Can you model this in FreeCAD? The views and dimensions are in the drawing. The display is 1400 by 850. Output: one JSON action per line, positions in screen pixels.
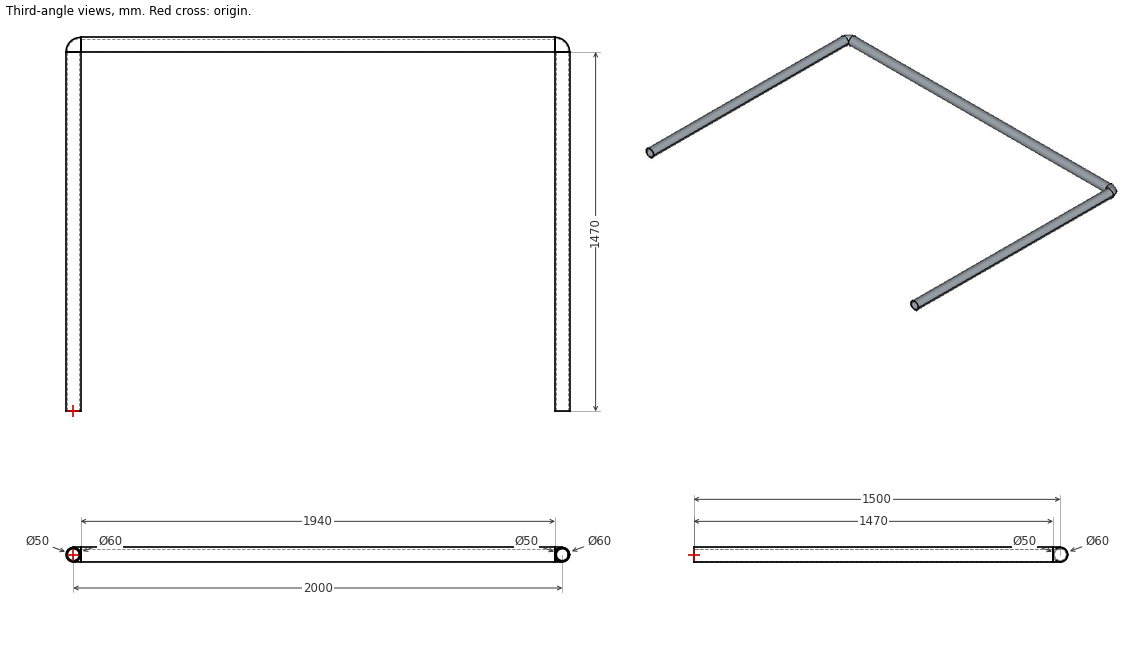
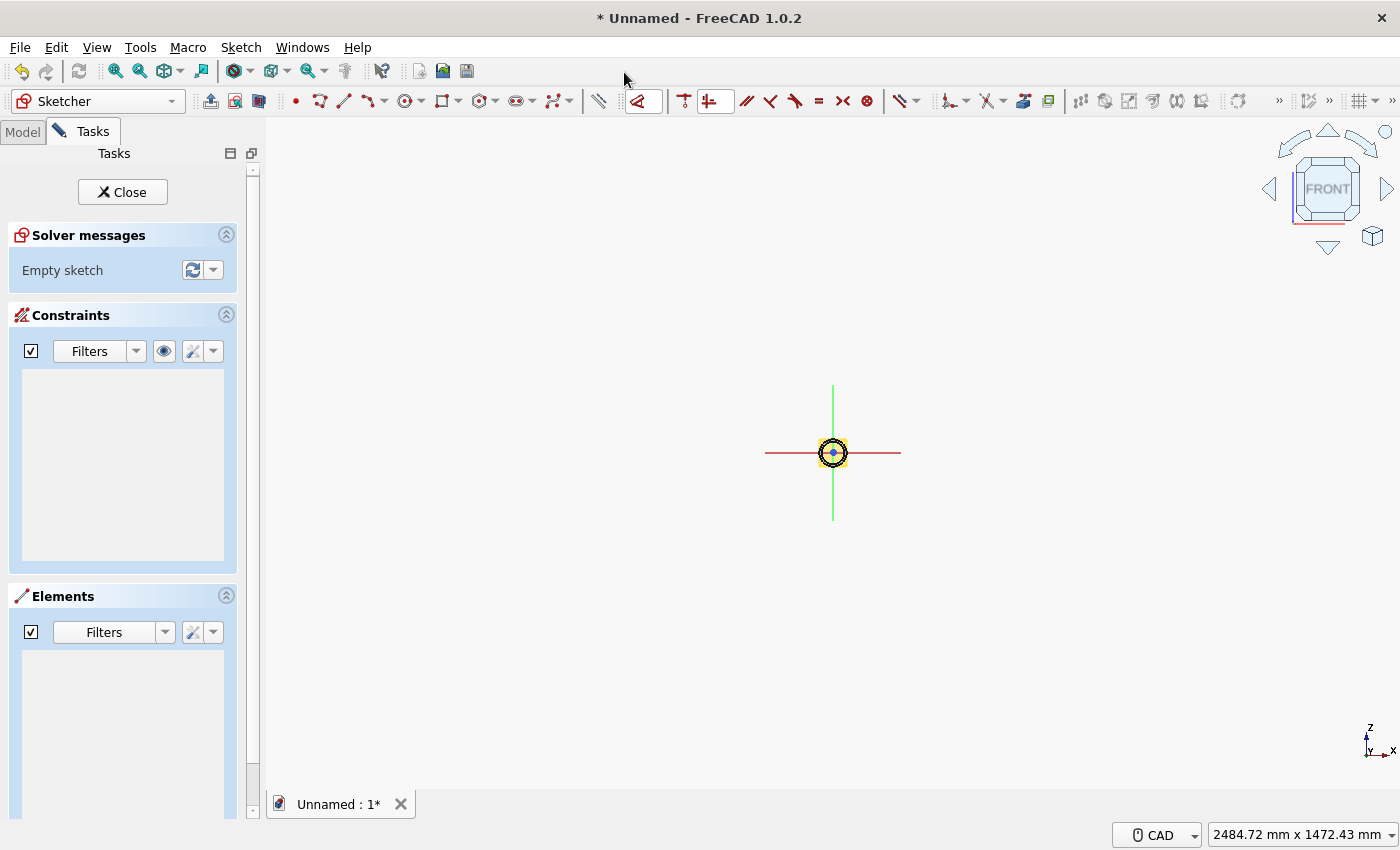
{"action": "scroll", "coordinate": [838, 453], "scroll_direction": "up", "scroll_amount": 13}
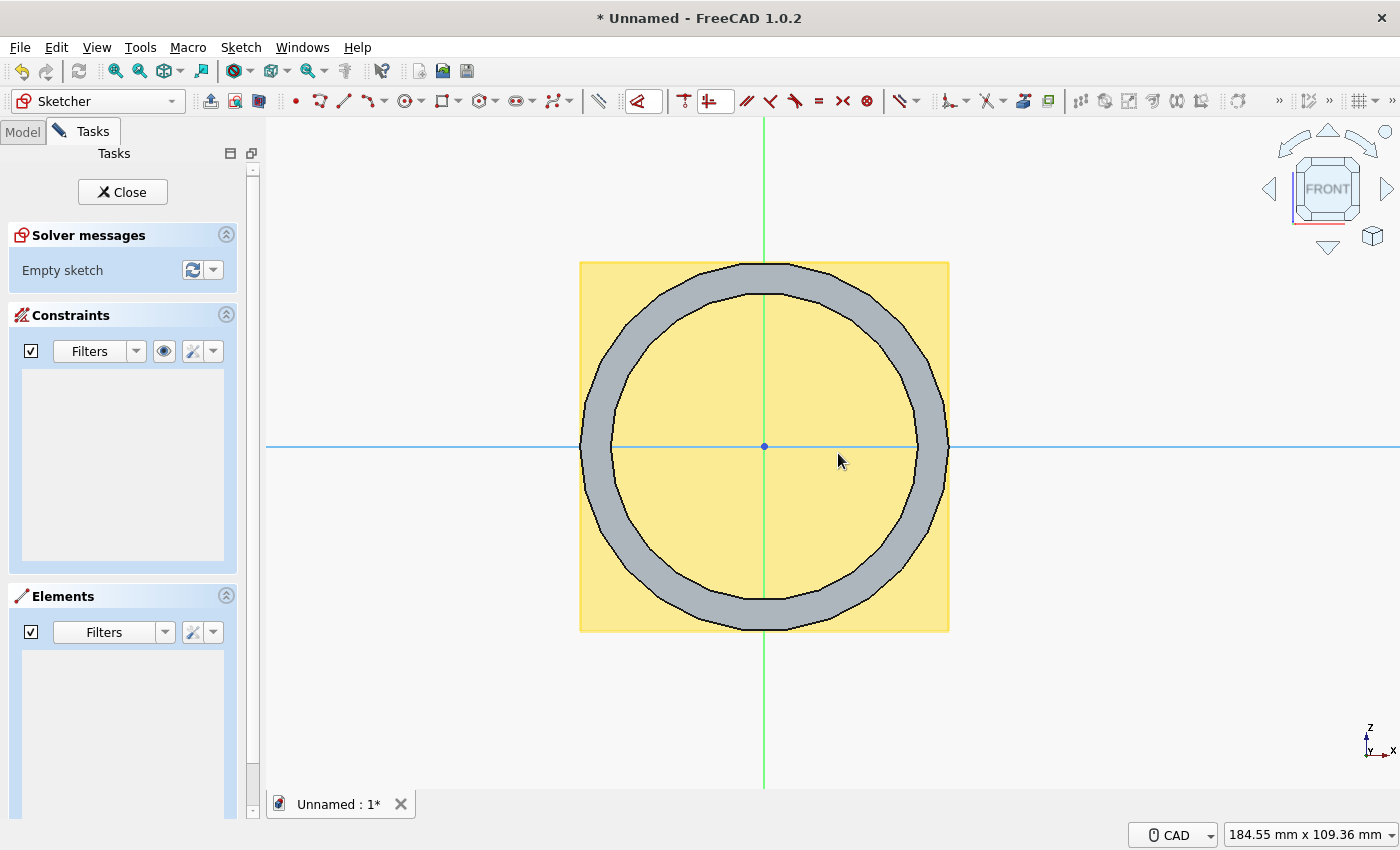
{"action": "left_click", "coordinate": [406, 102]}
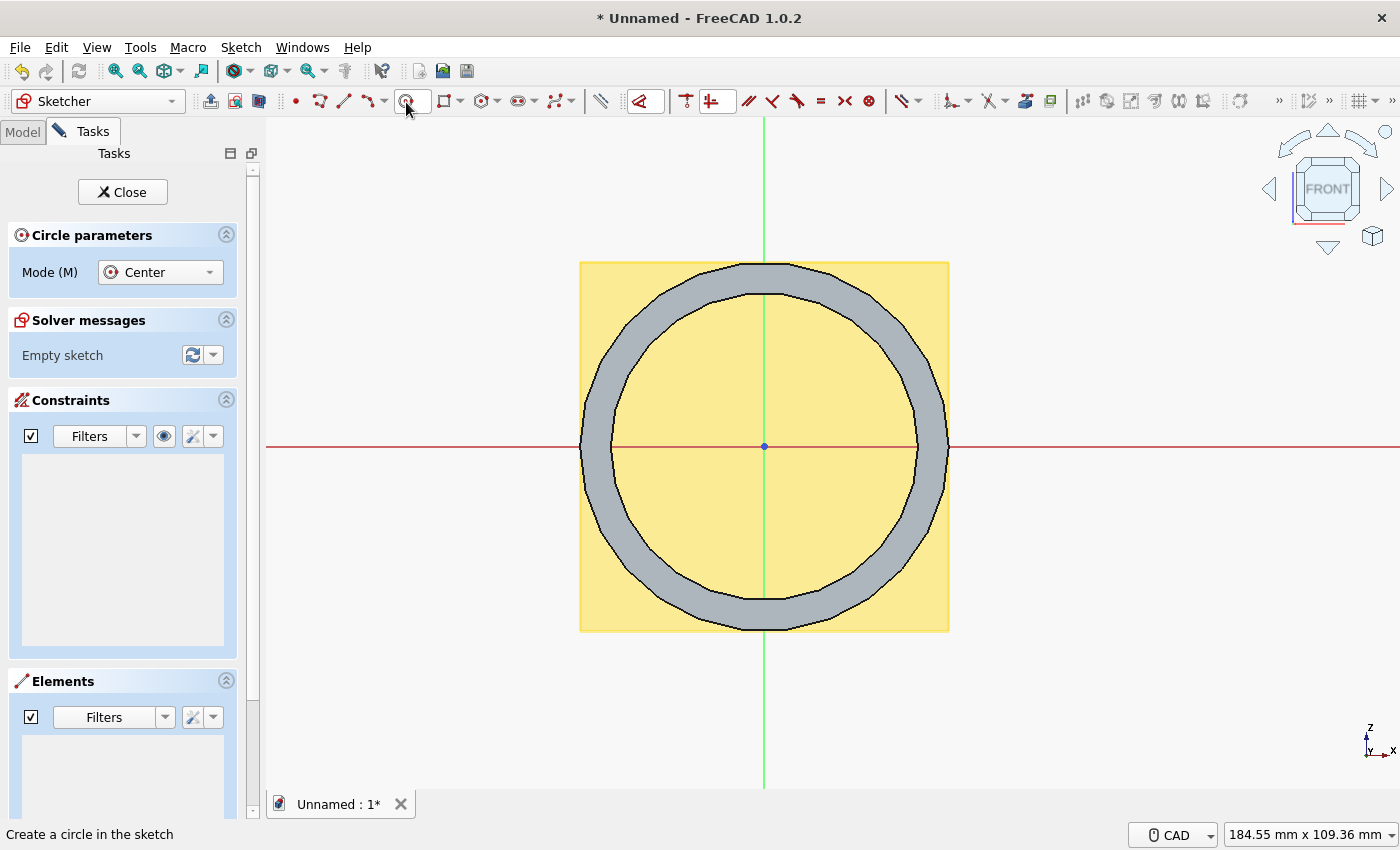
{"action": "left_click", "coordinate": [764, 447]}
{"action": "mouse_move", "coordinate": [895, 316]}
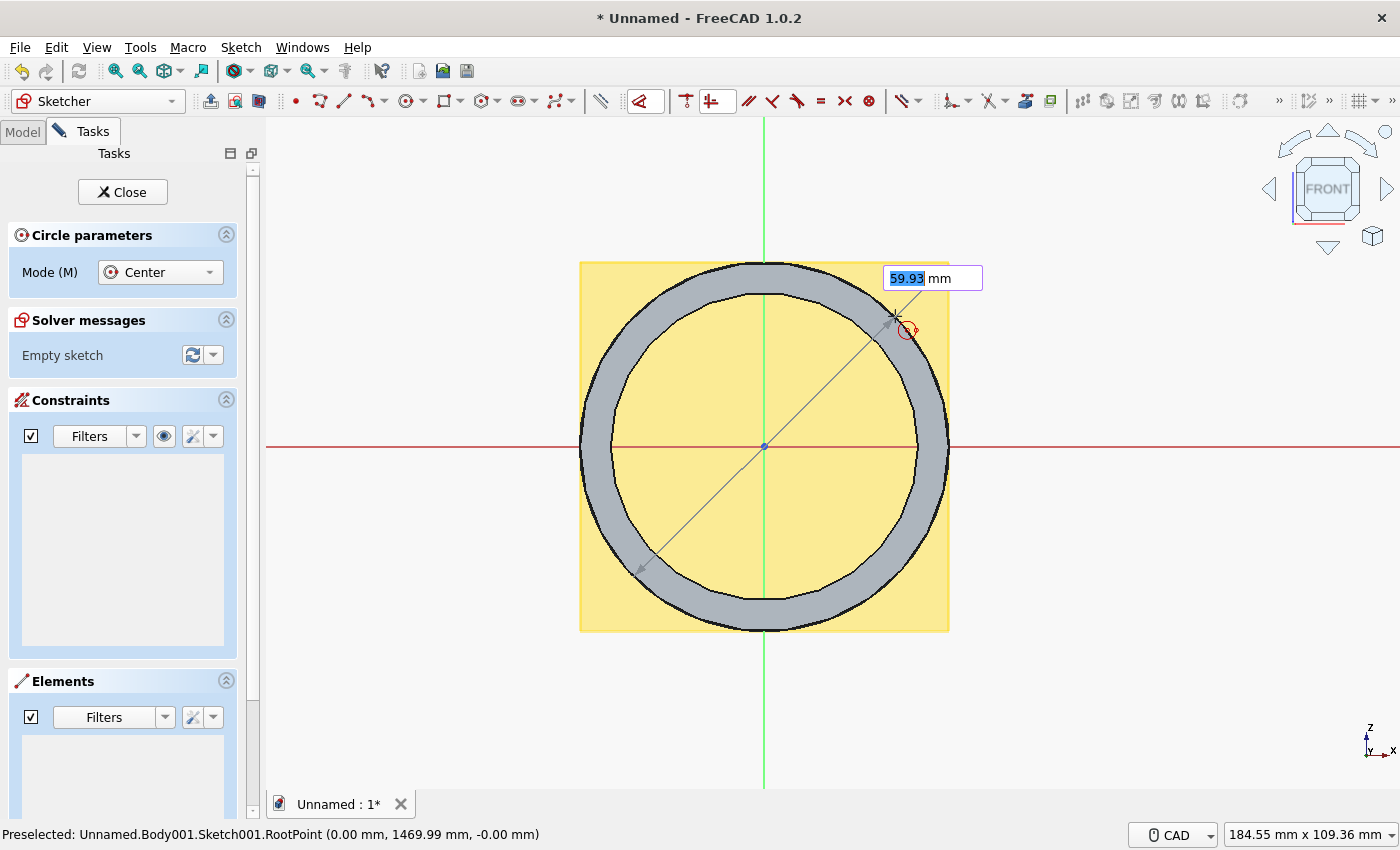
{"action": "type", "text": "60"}
{"action": "key", "text": "Return"}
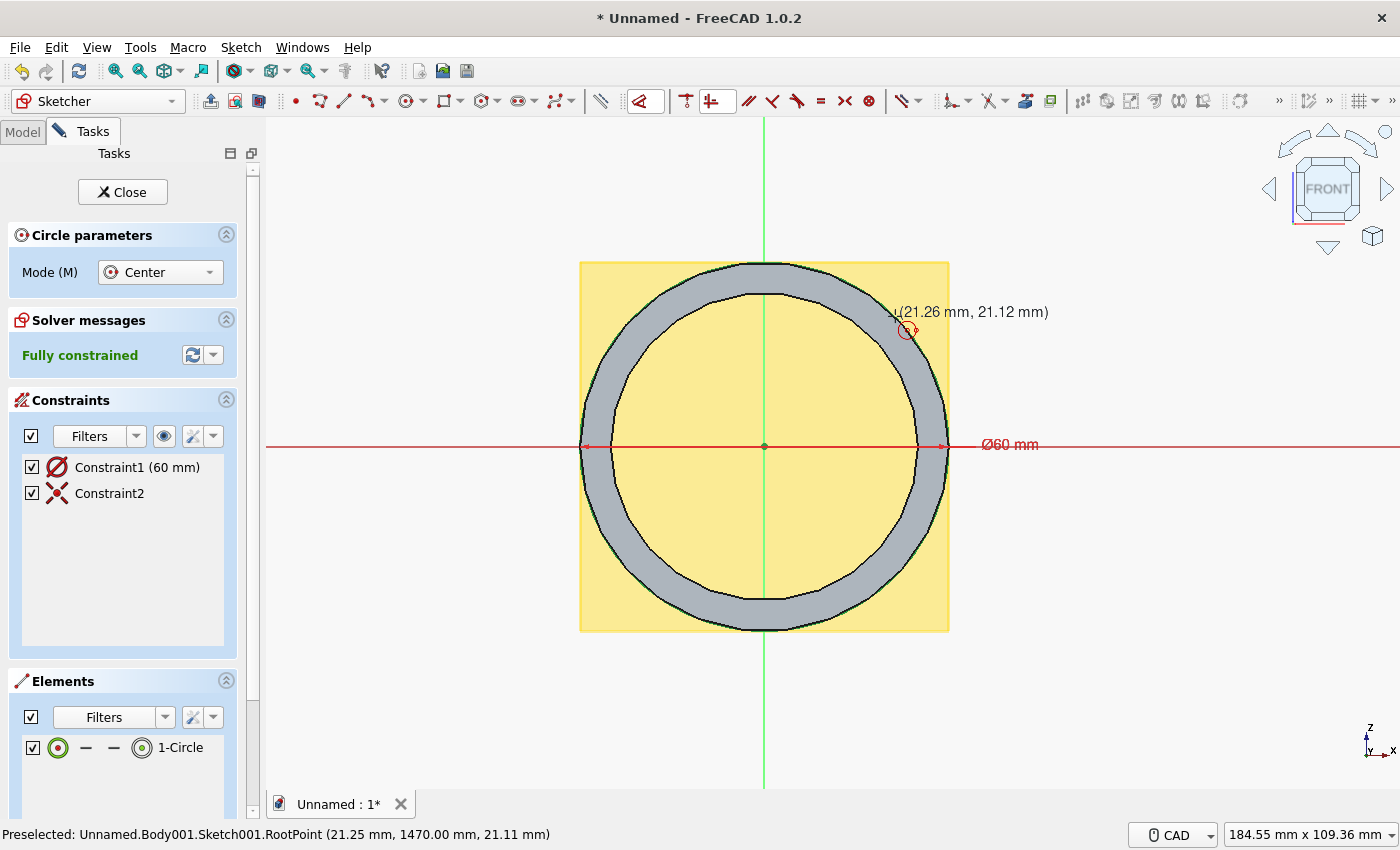
{"action": "left_click", "coordinate": [764, 447]}
{"action": "mouse_move", "coordinate": [873, 338]}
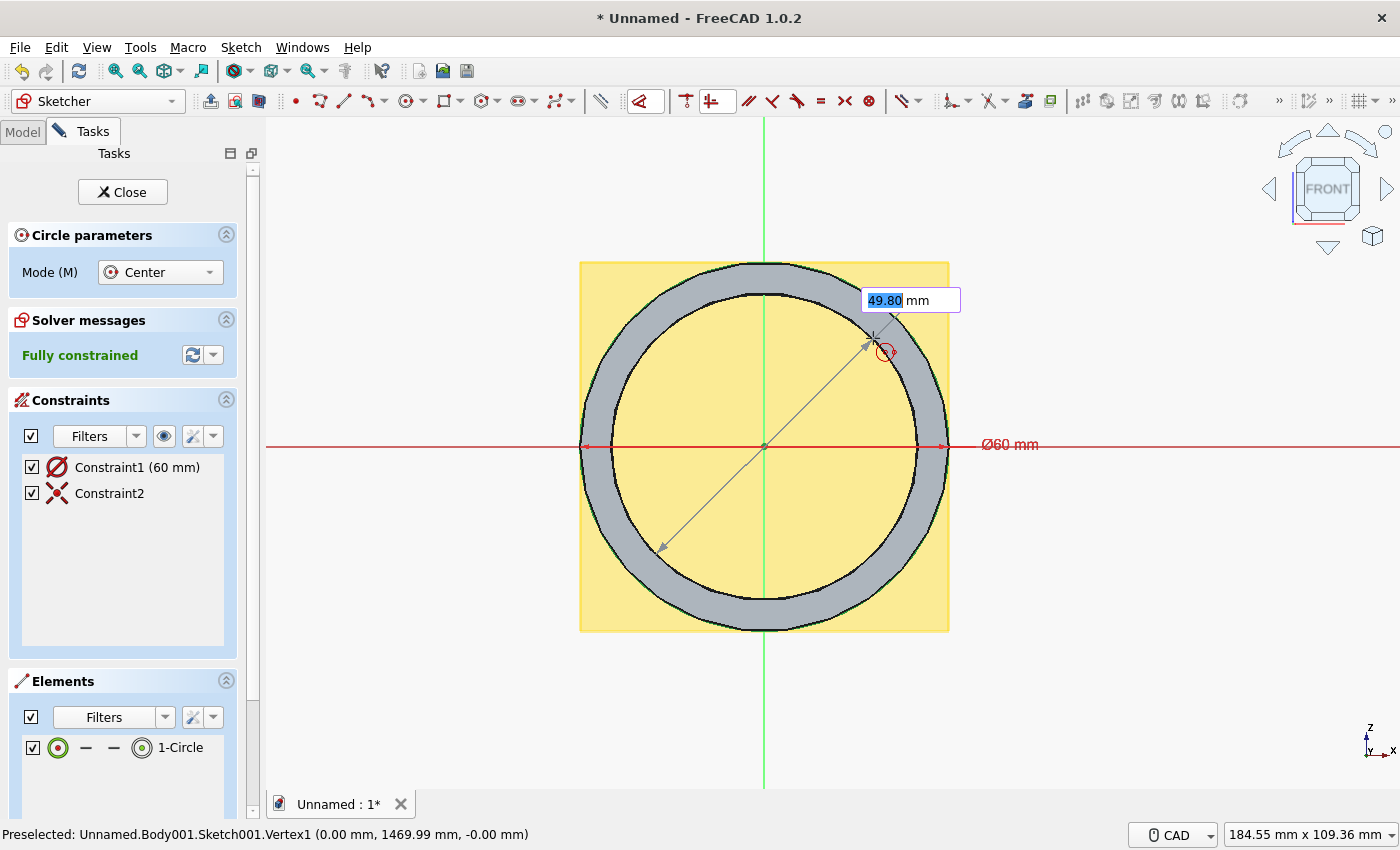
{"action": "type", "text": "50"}
{"action": "key", "text": "Return"}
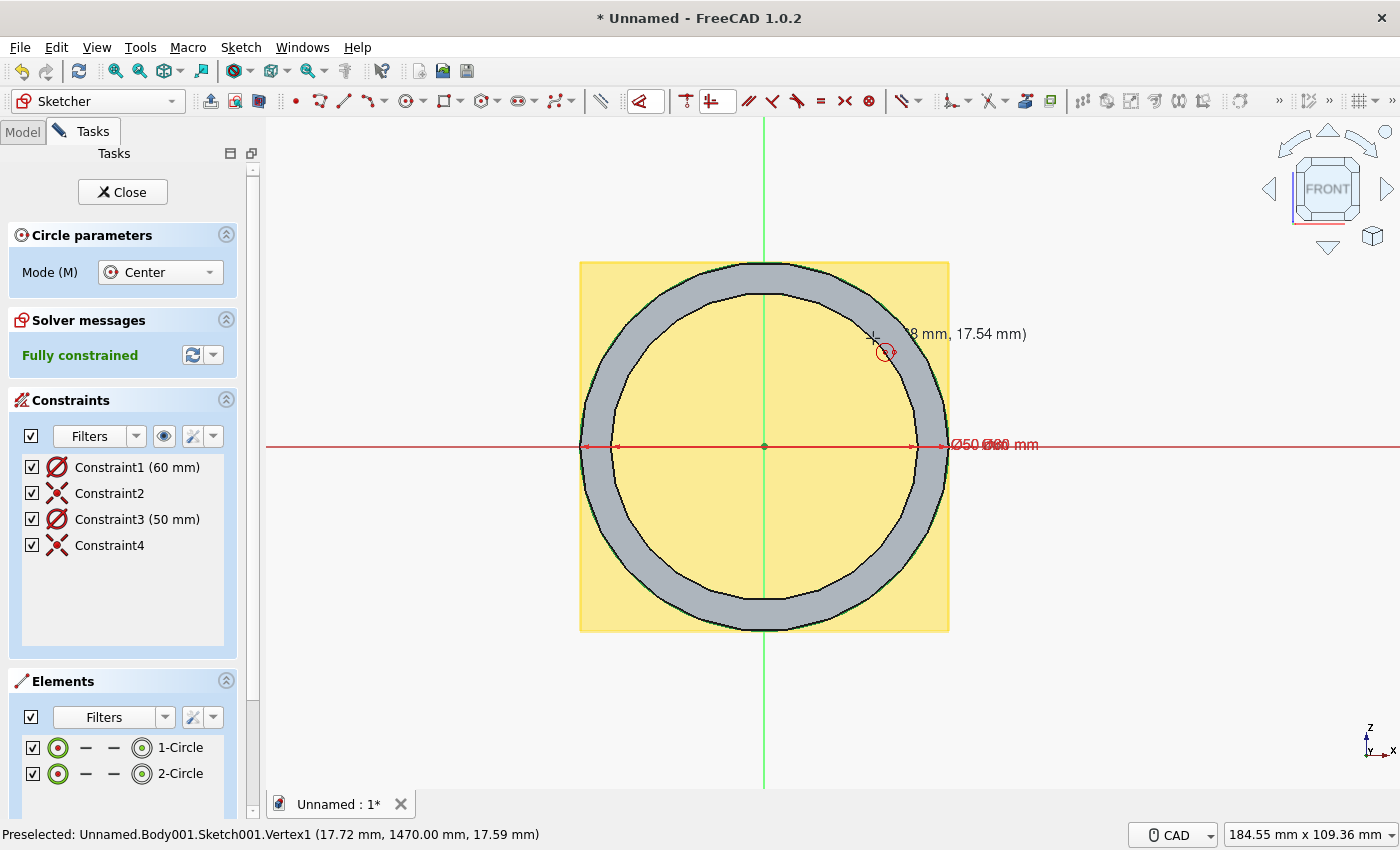
{"action": "left_click", "coordinate": [344, 102]}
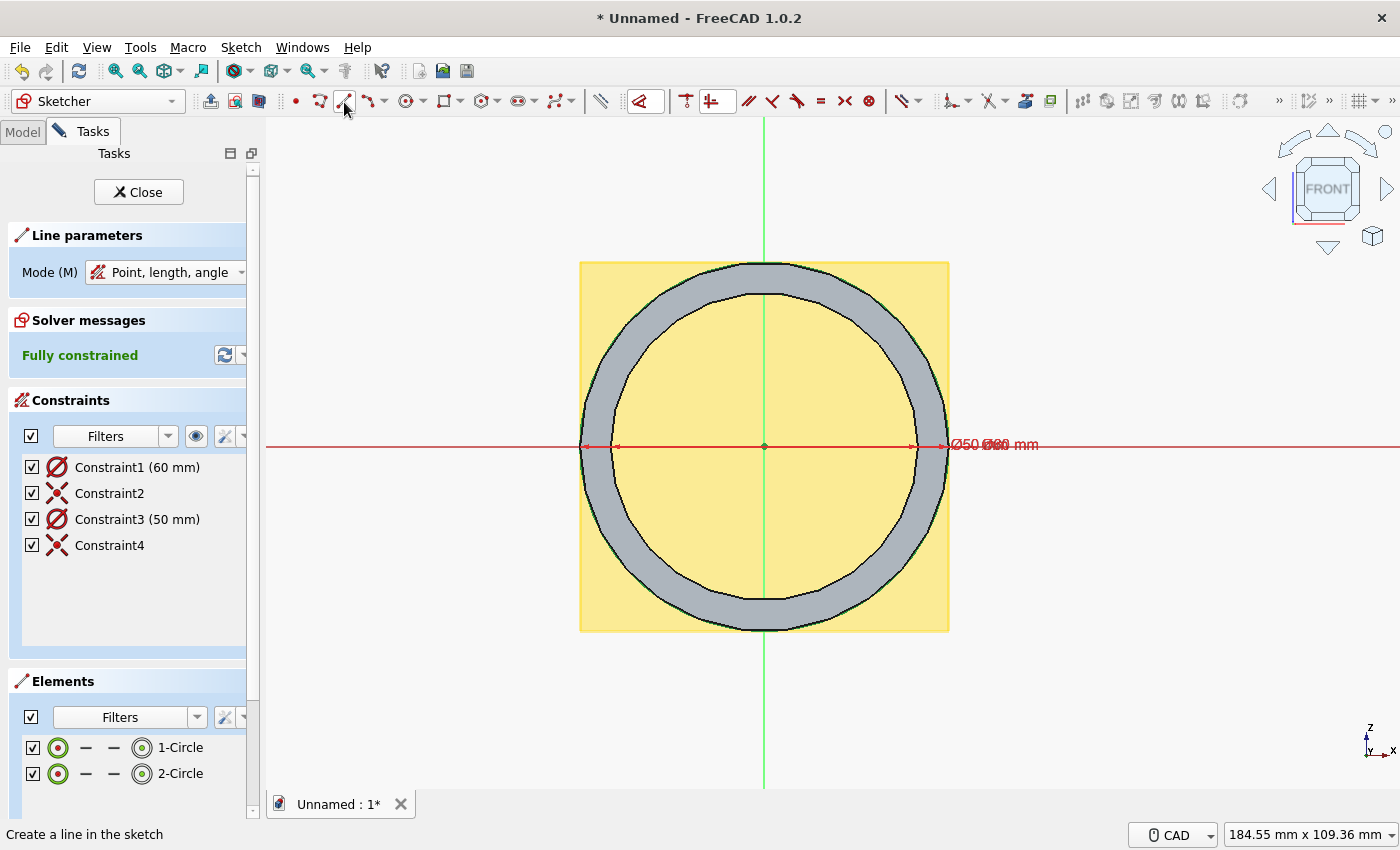
{"action": "left_click", "coordinate": [949, 226]}
{"action": "left_click", "coordinate": [949, 668]}
{"action": "key", "text": "Escape"}